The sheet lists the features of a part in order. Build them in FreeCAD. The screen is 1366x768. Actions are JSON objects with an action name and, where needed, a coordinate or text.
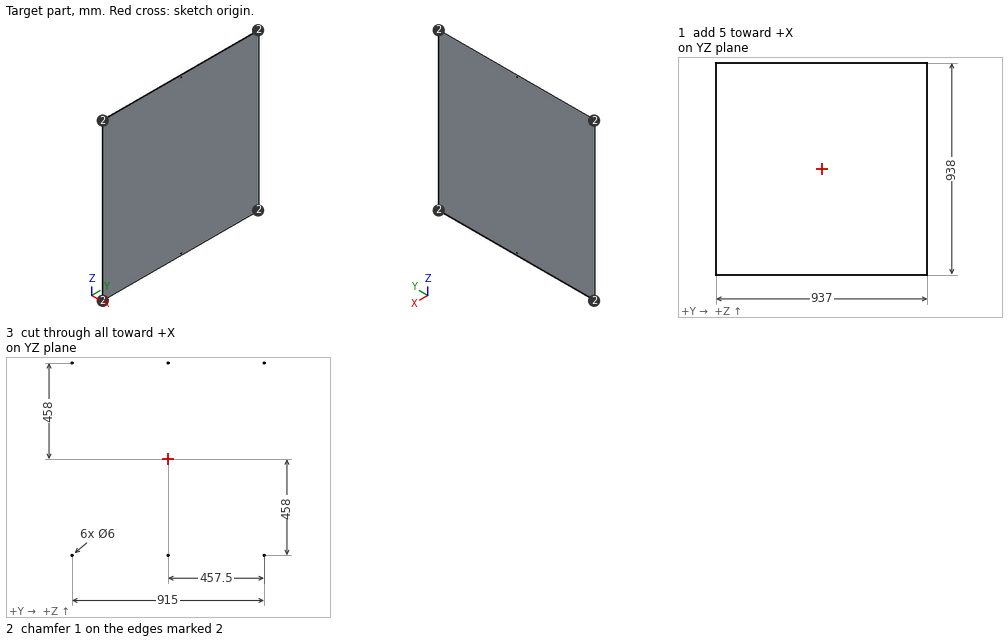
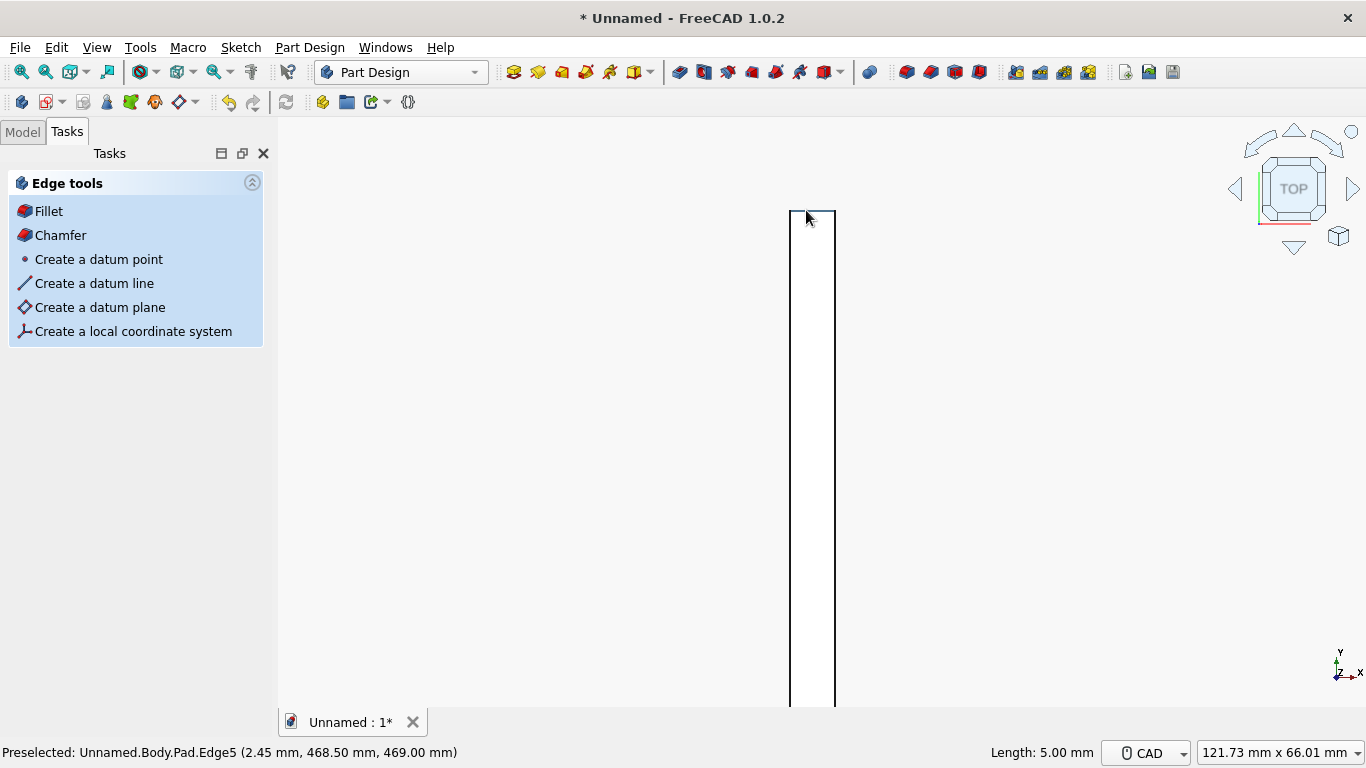
{"action": "left_click", "coordinate": [22, 72]}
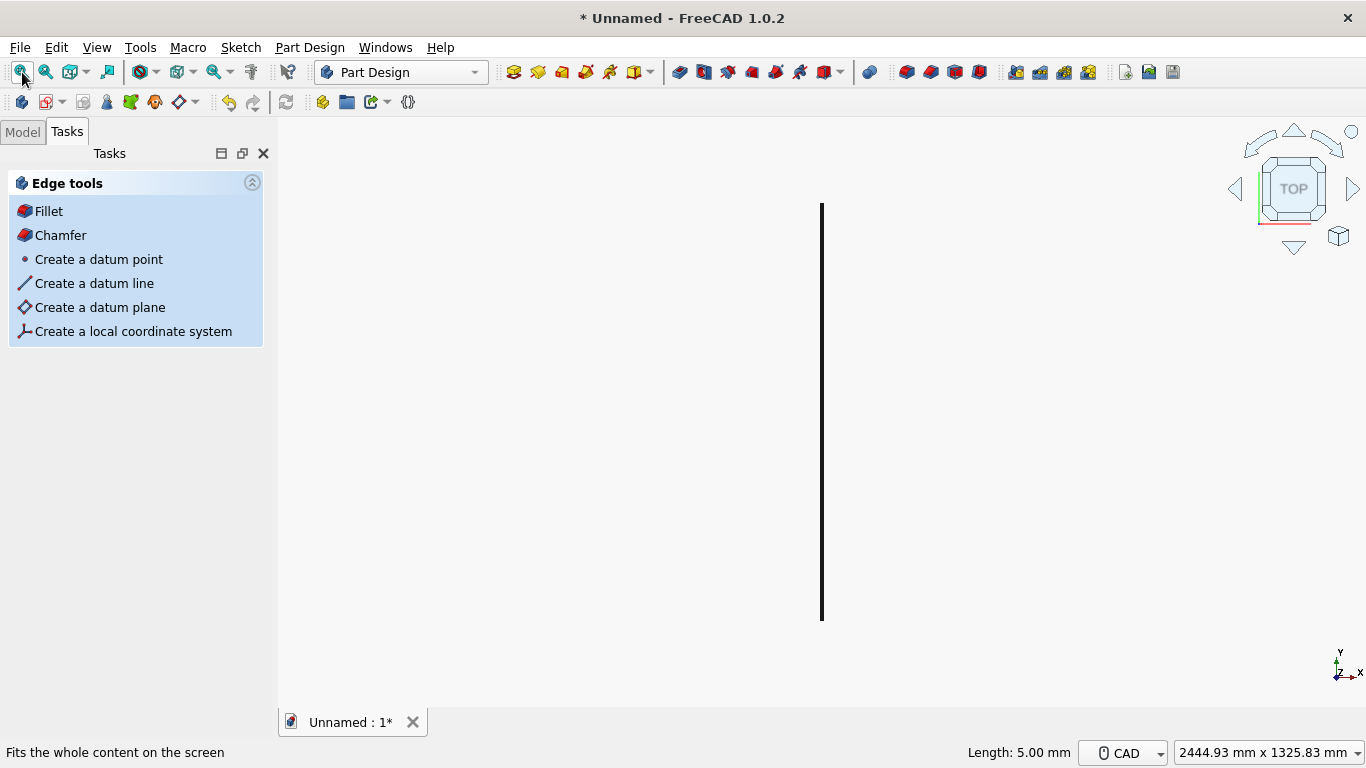
{"action": "key", "text": "1"}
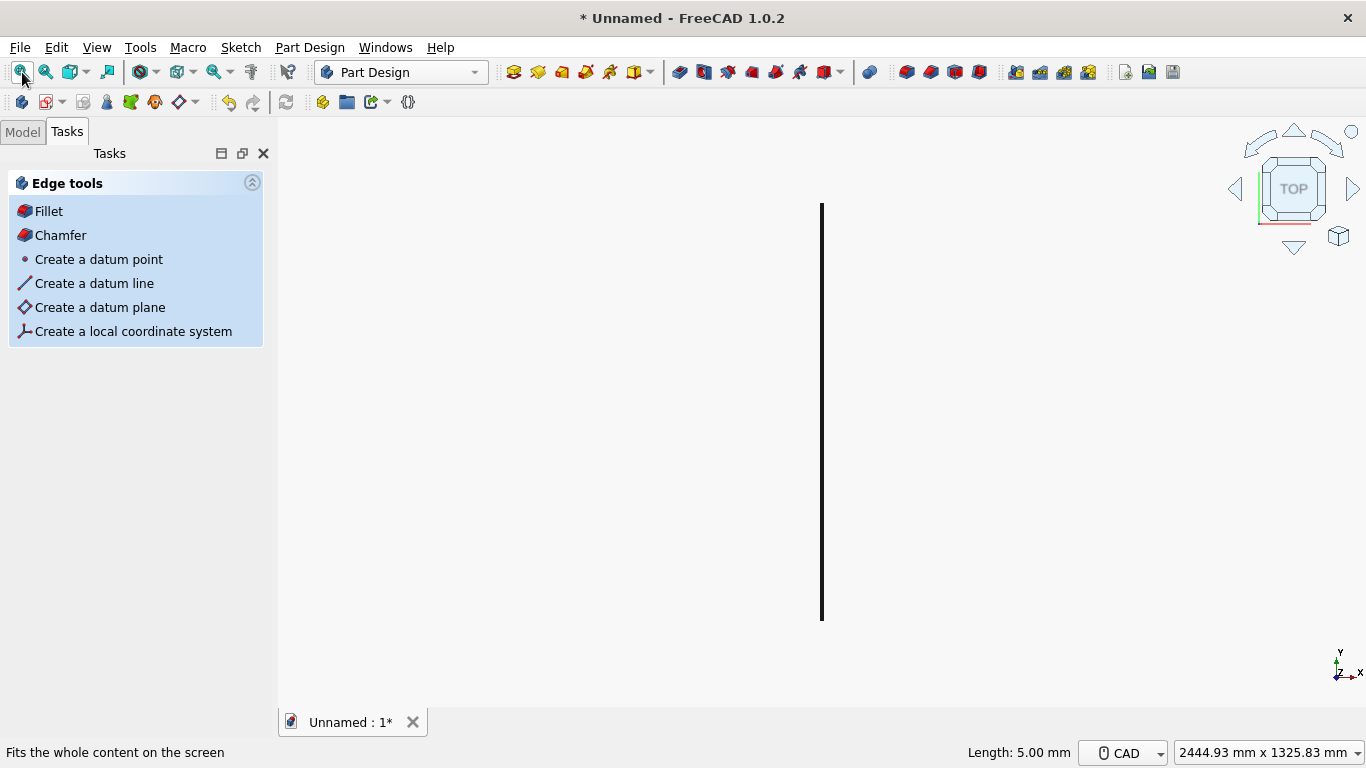
{"action": "scroll", "coordinate": [822, 620], "scroll_direction": "up", "scroll_amount": 15}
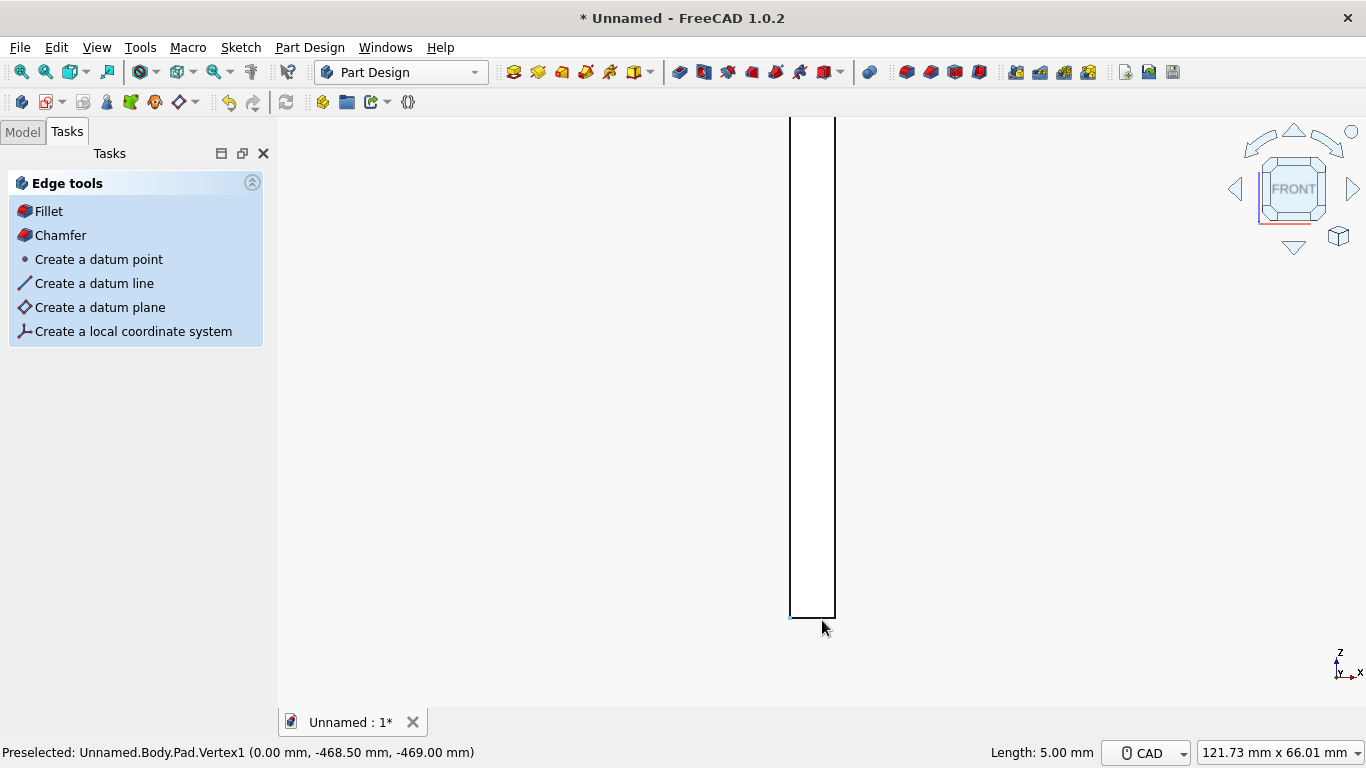
{"action": "left_click", "coordinate": [812, 617], "text": "ctrl"}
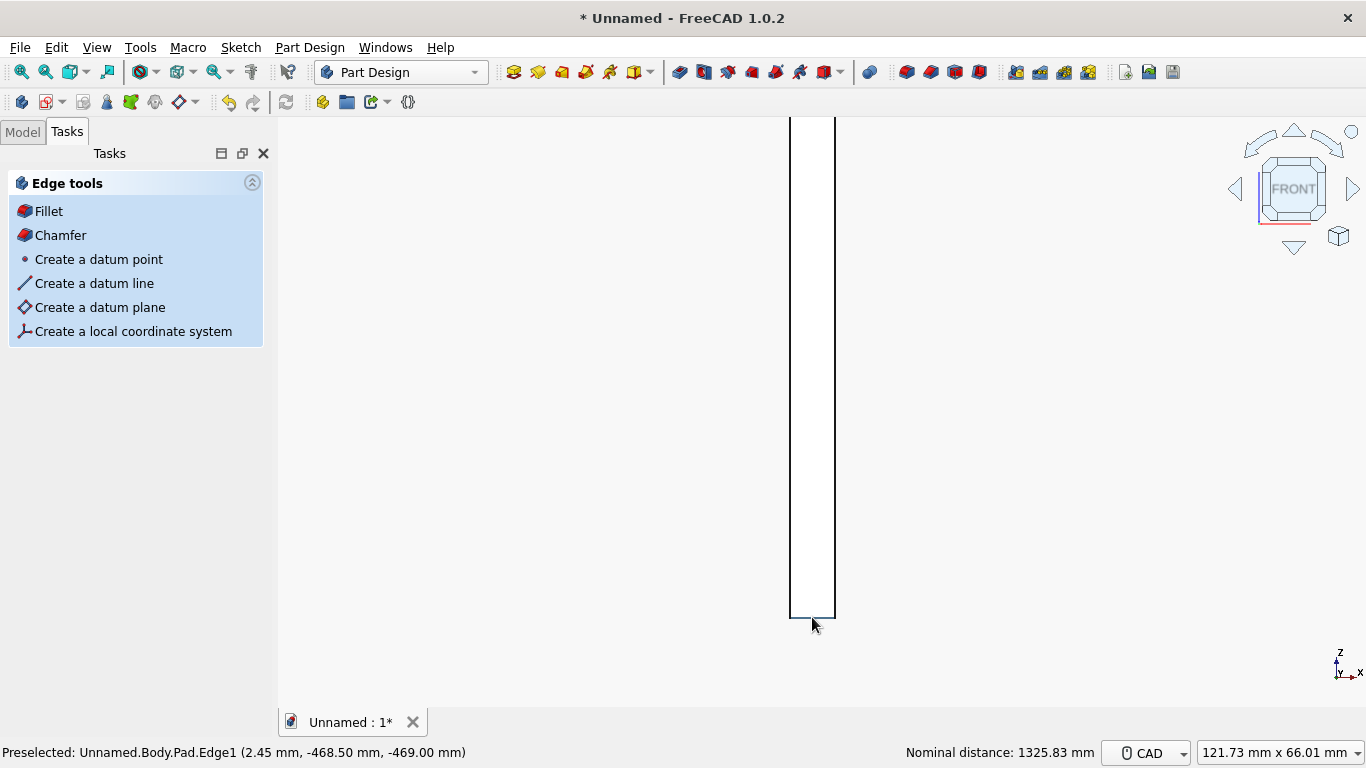
{"action": "left_click", "coordinate": [22, 72]}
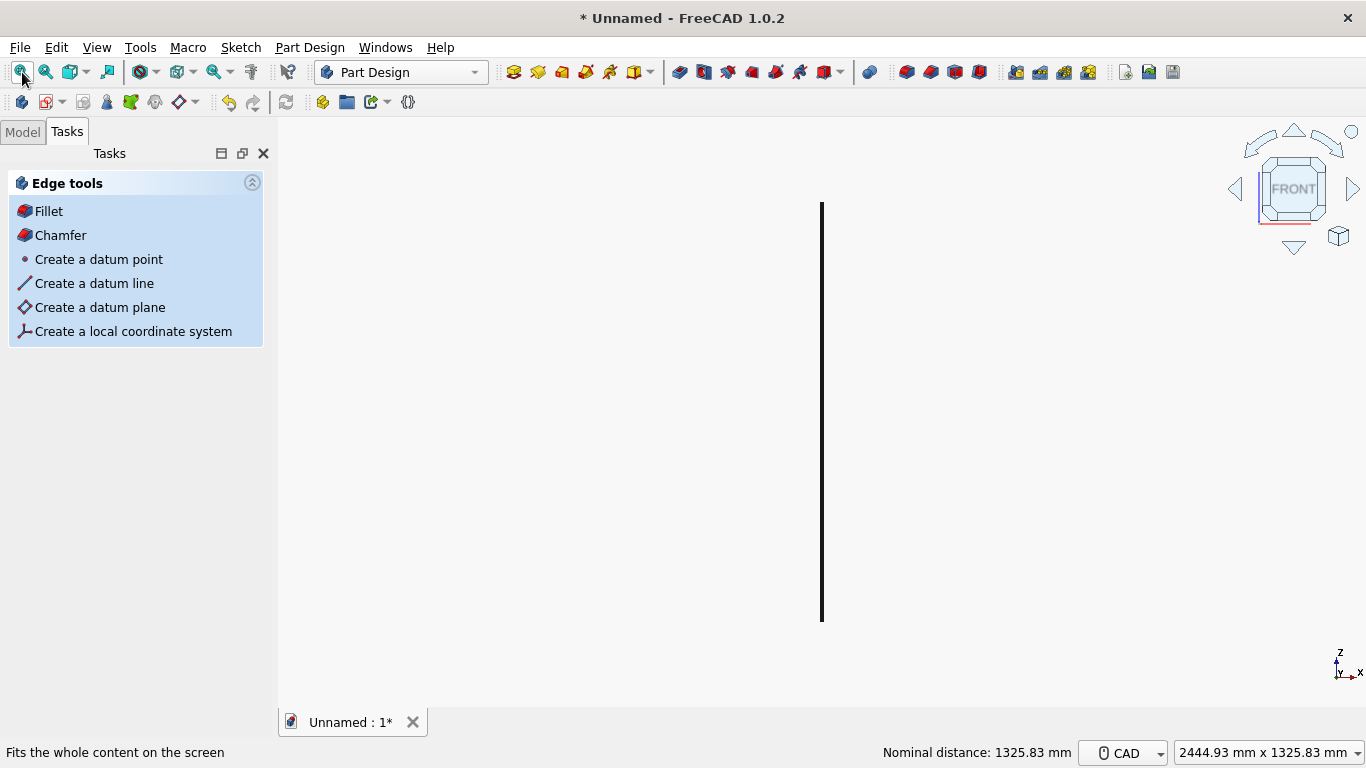
{"action": "key", "text": "3"}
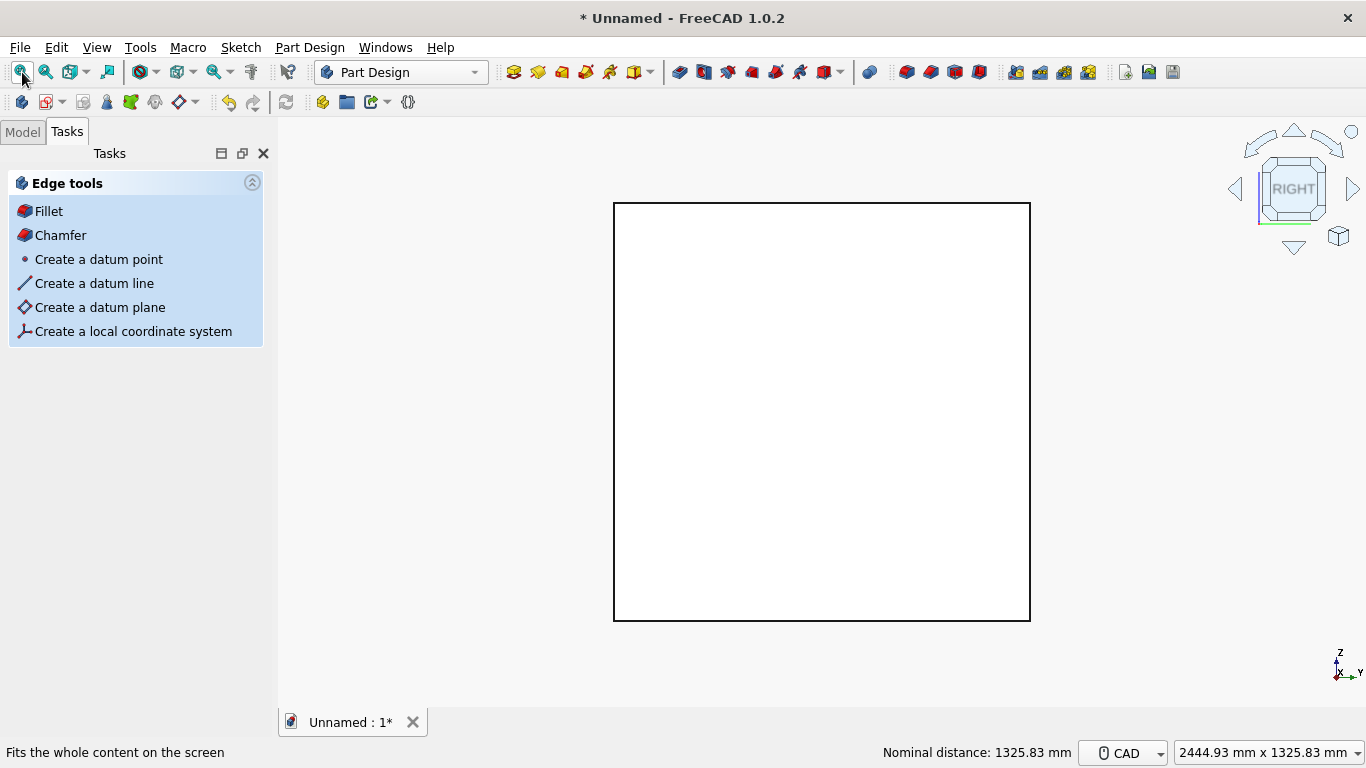
{"action": "scroll", "coordinate": [1030, 620], "scroll_direction": "up", "scroll_amount": 15}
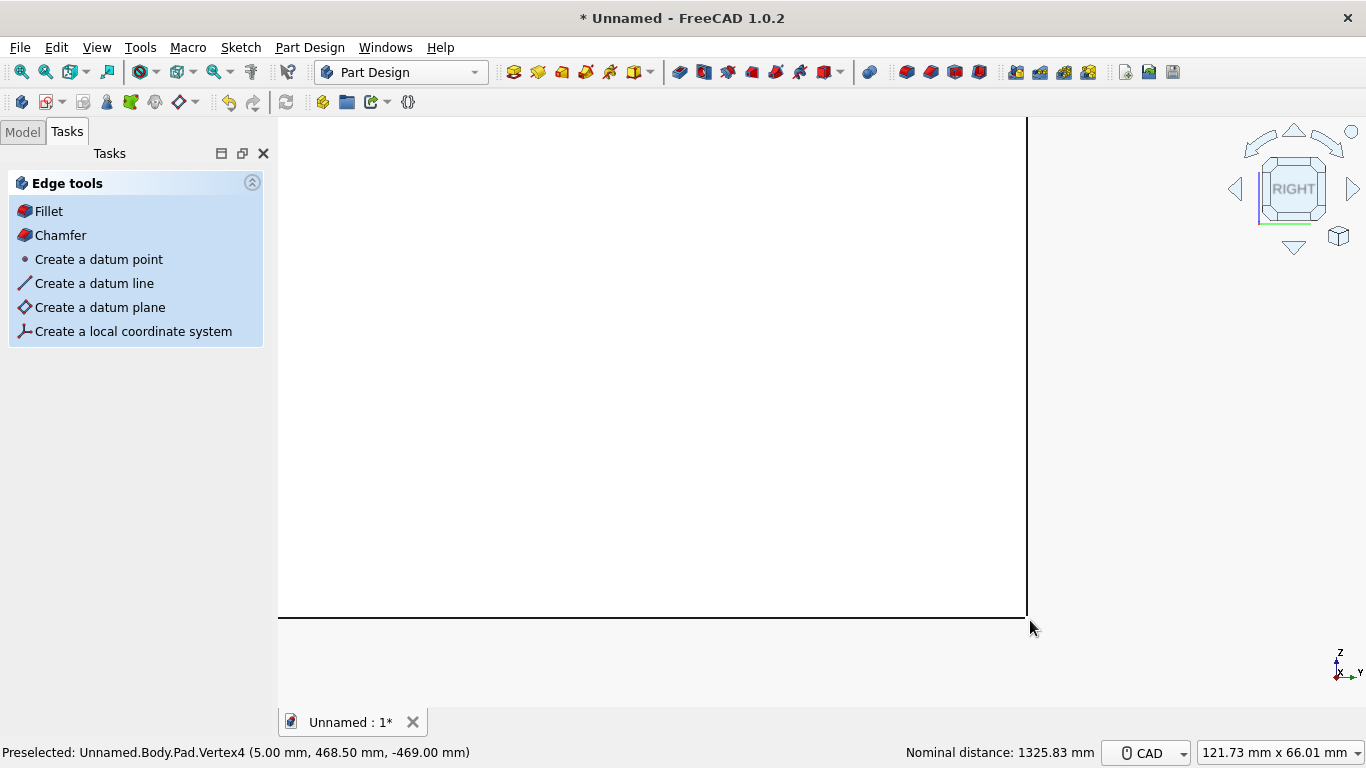
{"action": "left_click", "coordinate": [22, 72]}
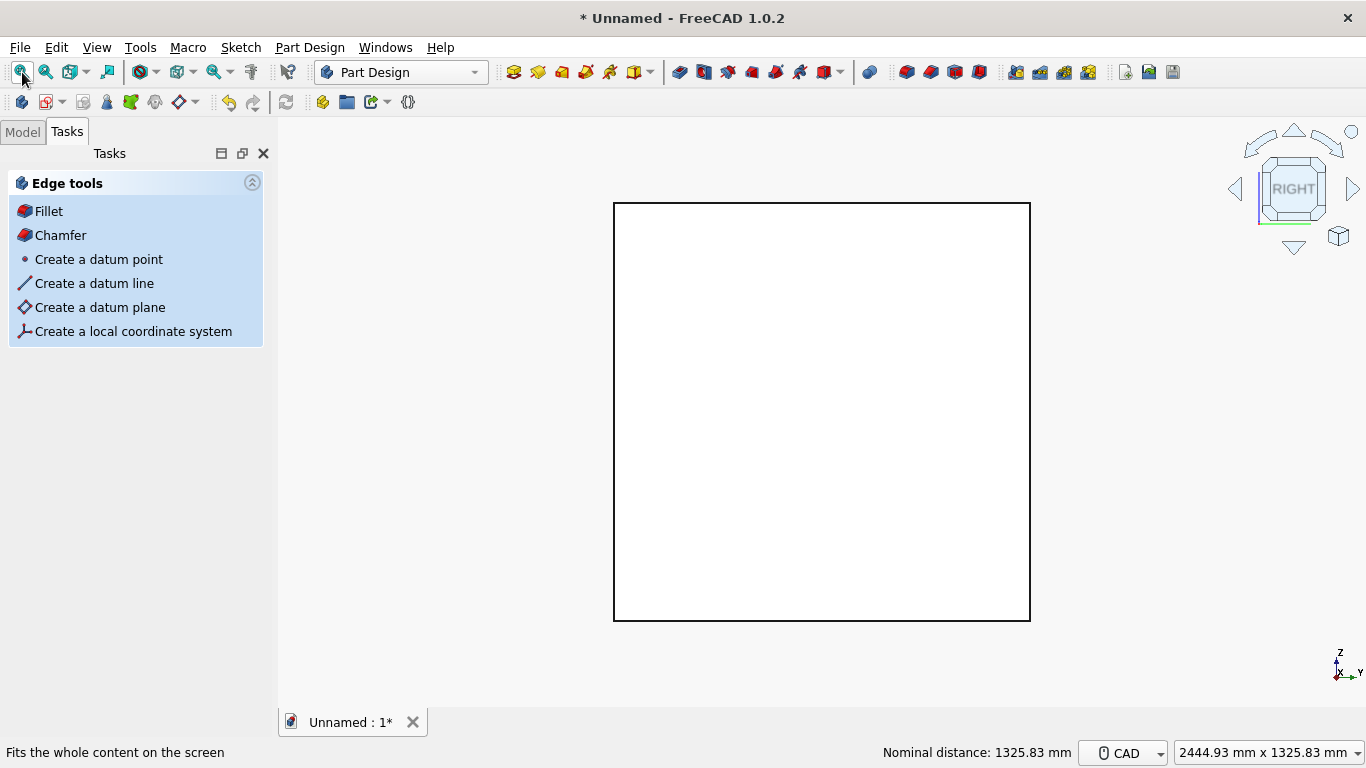
{"action": "key", "text": "5"}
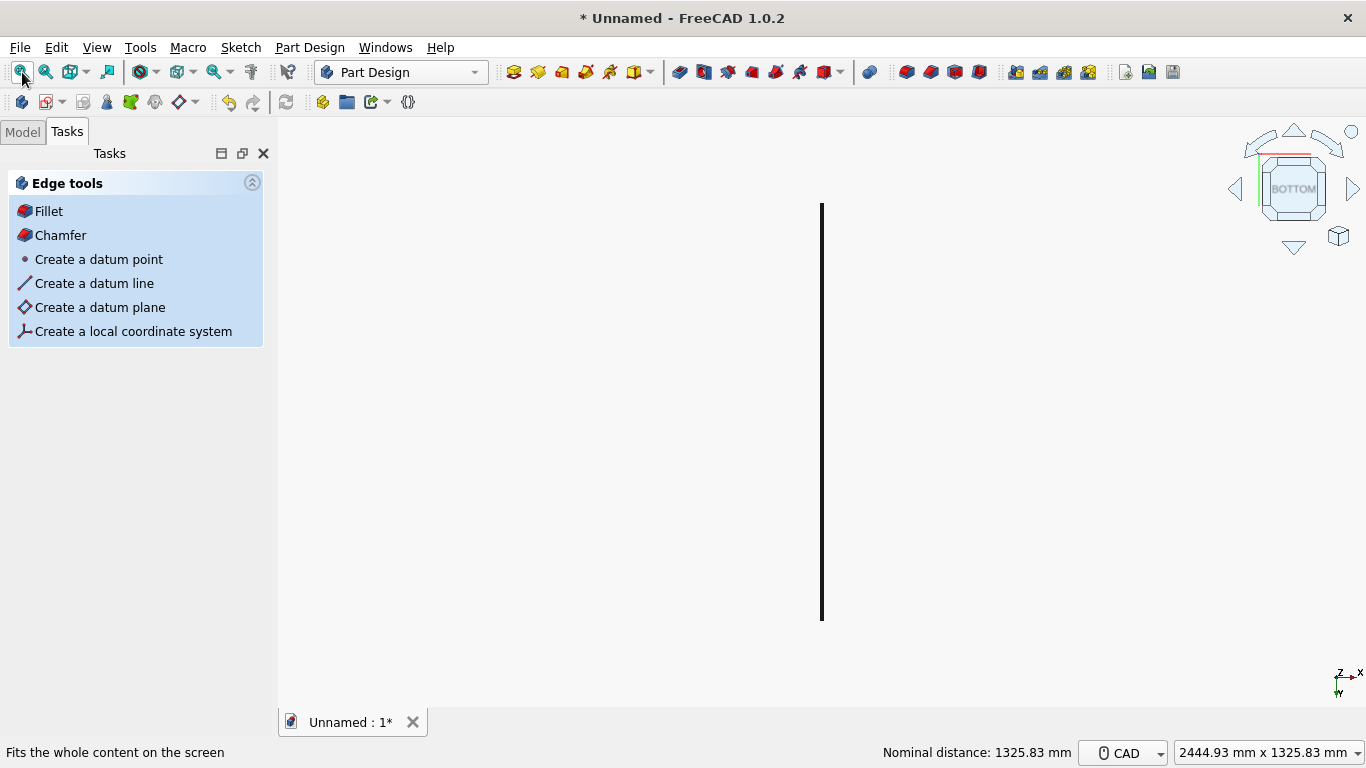
{"action": "scroll", "coordinate": [822, 619], "scroll_direction": "up", "scroll_amount": 15}